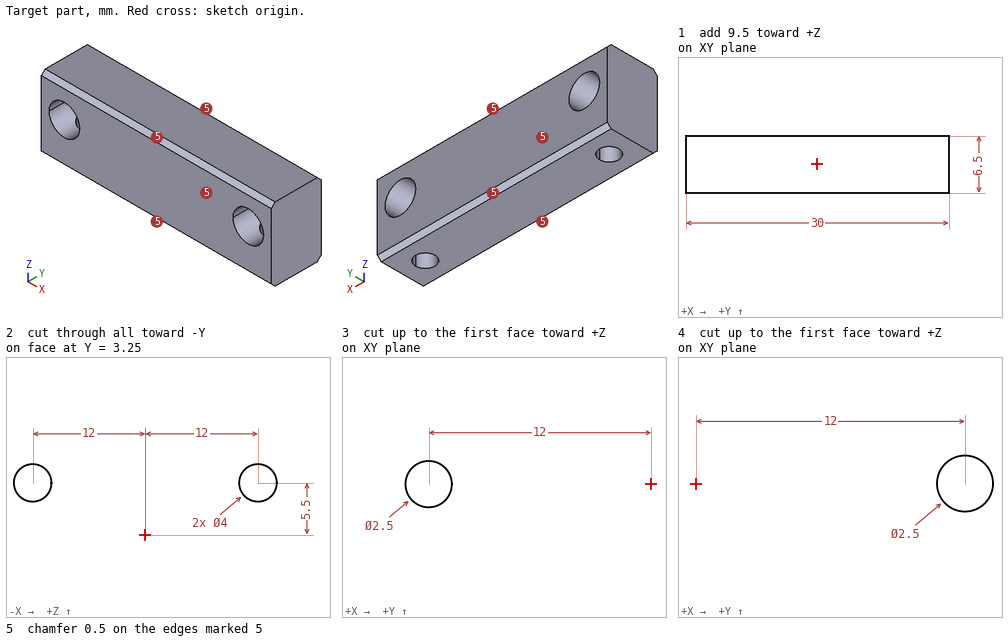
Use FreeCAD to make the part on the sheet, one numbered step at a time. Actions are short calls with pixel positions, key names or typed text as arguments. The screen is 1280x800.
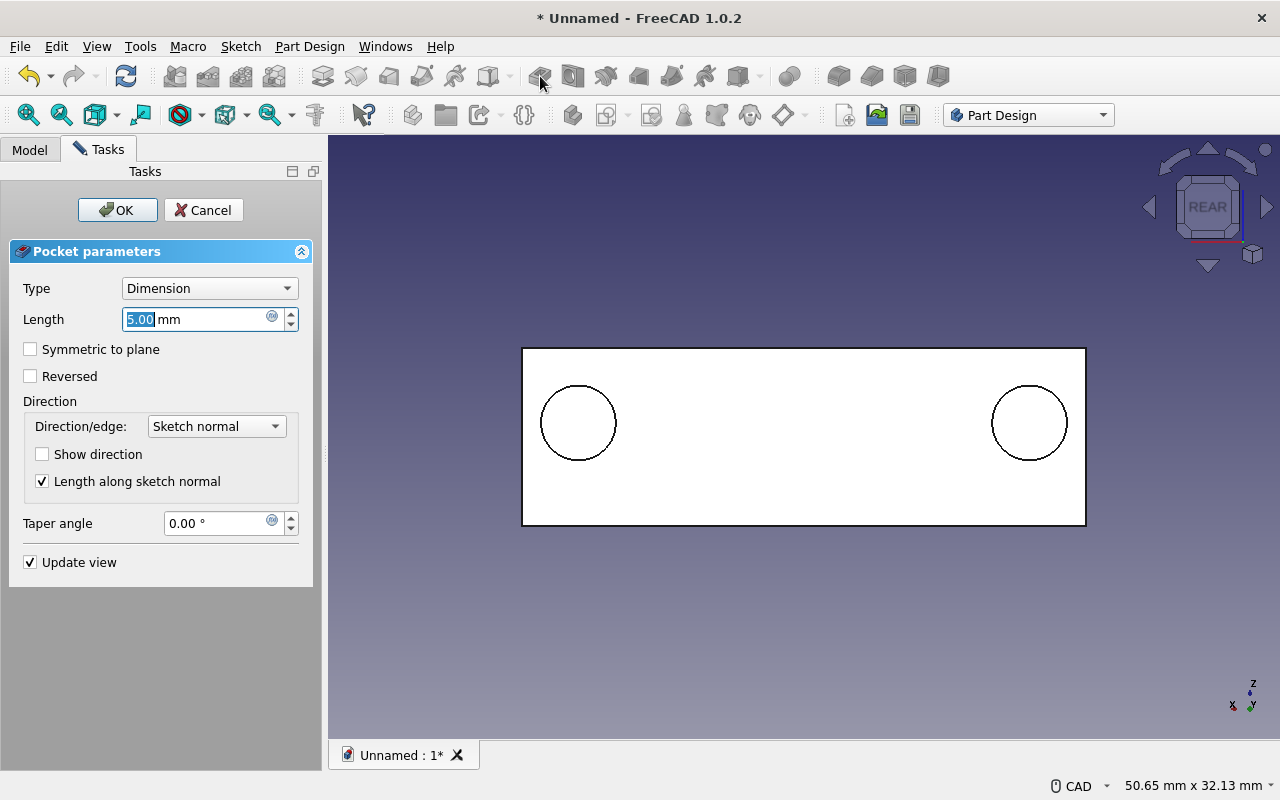
click(210, 288)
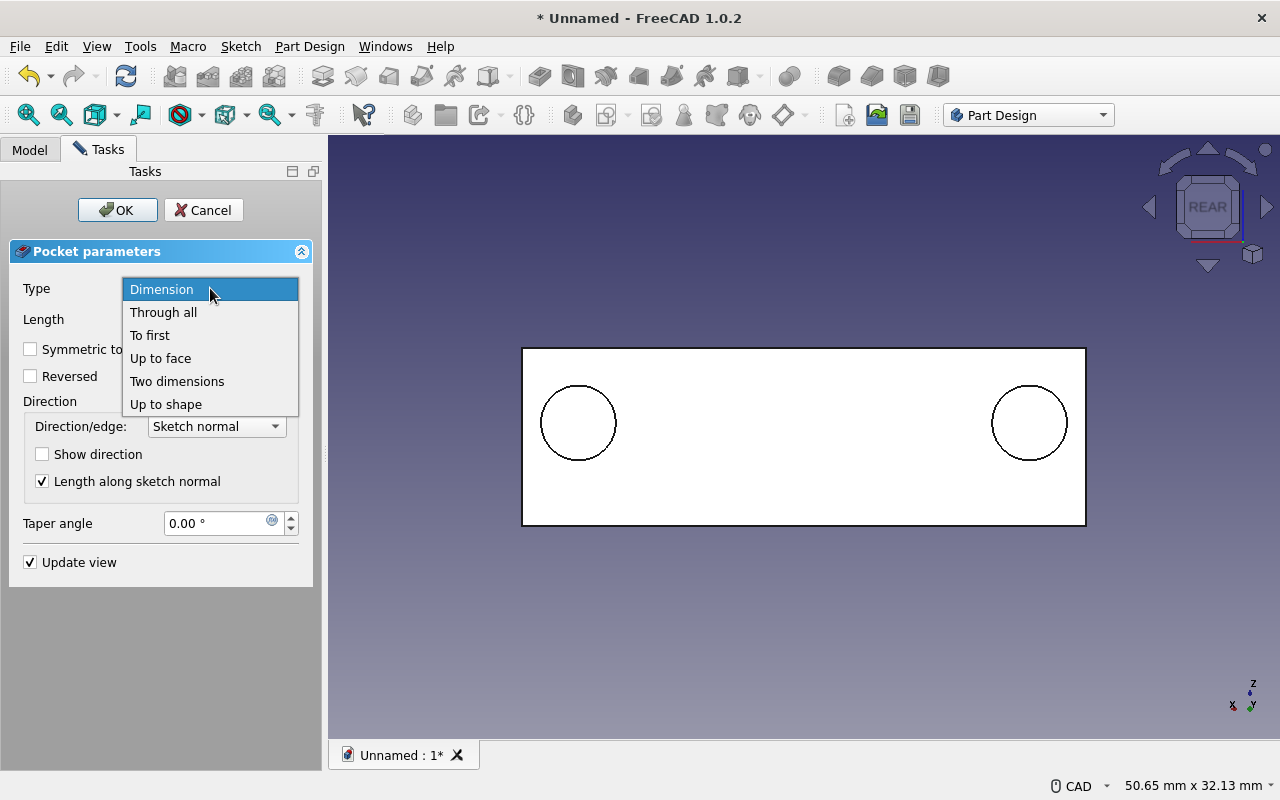
click(208, 312)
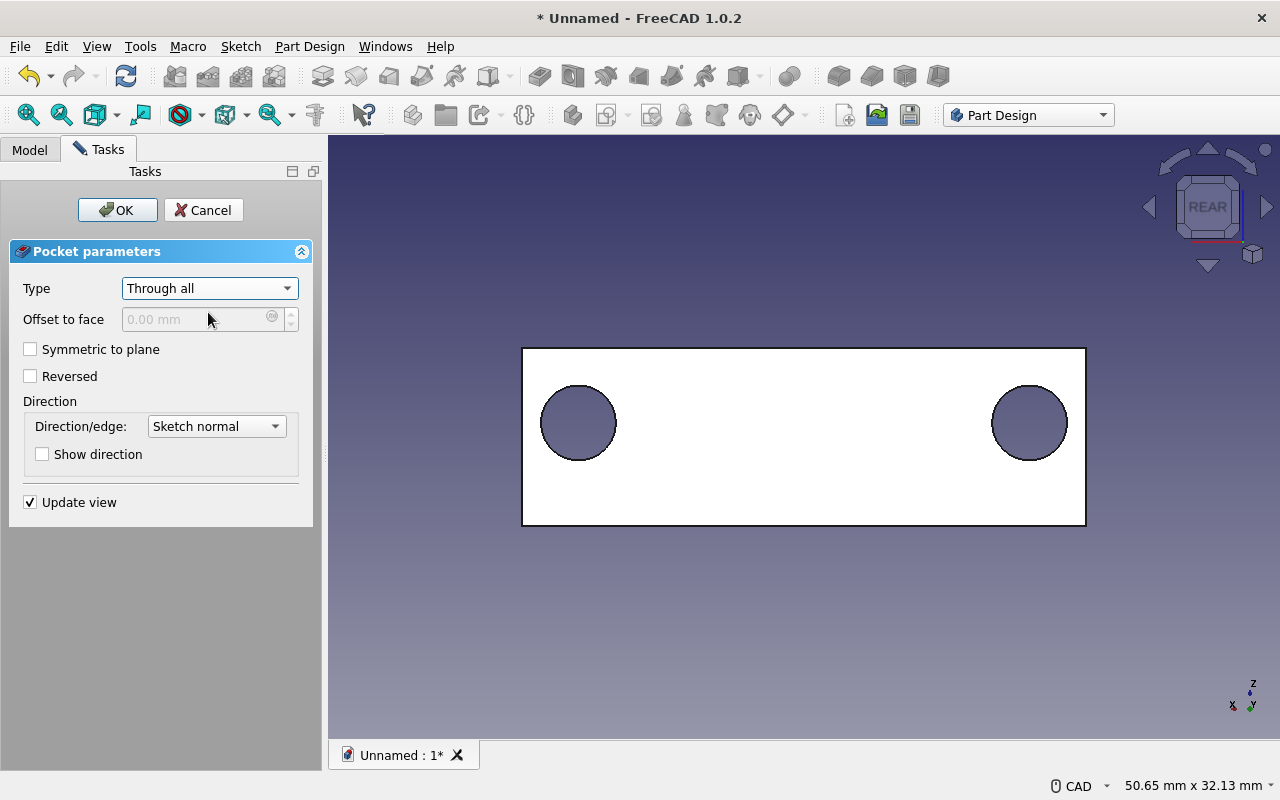
click(118, 210)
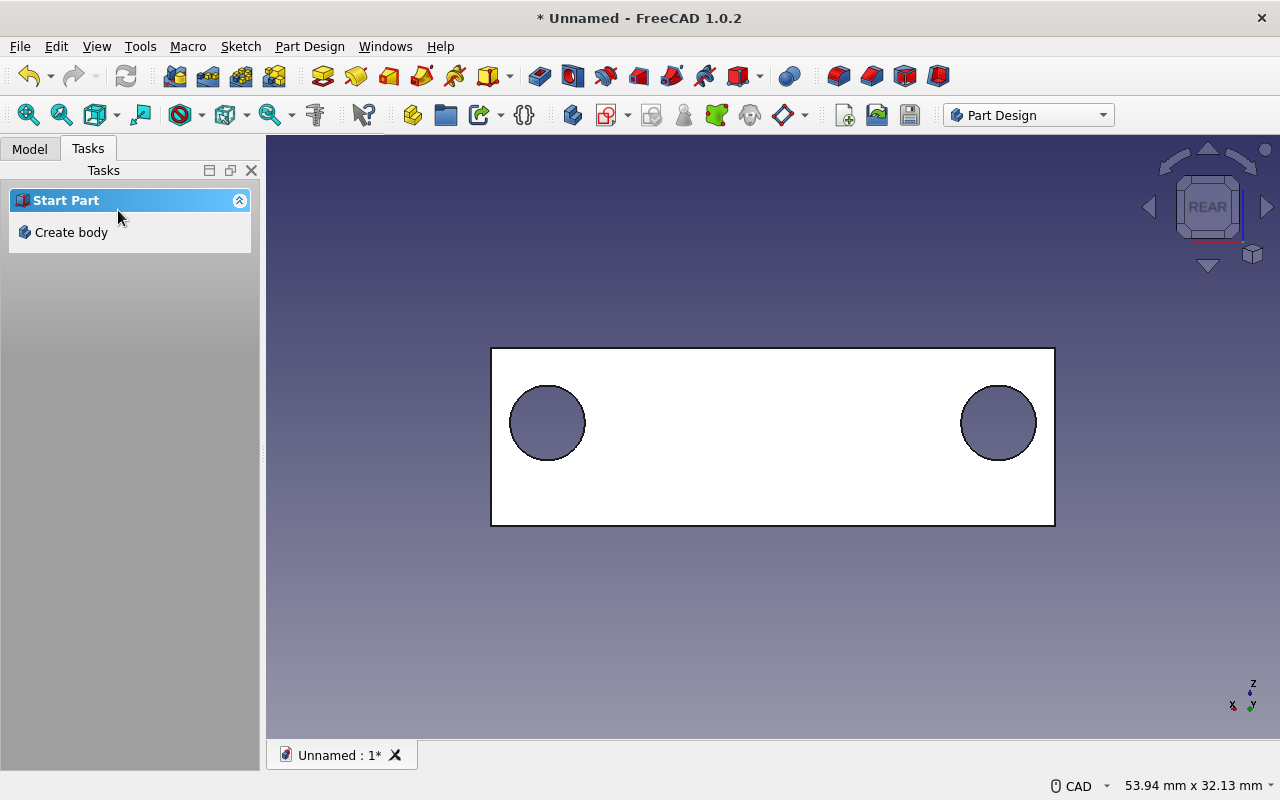
click(606, 116)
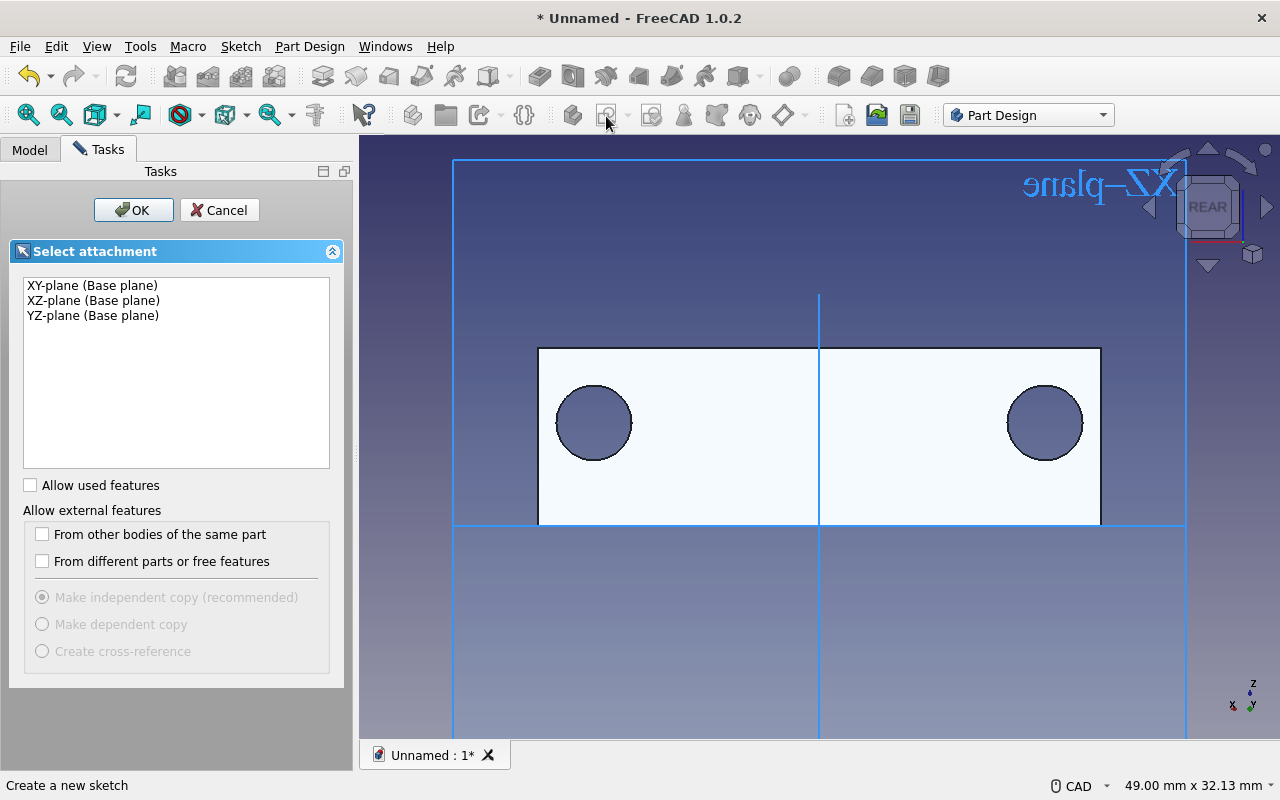
click(84, 286)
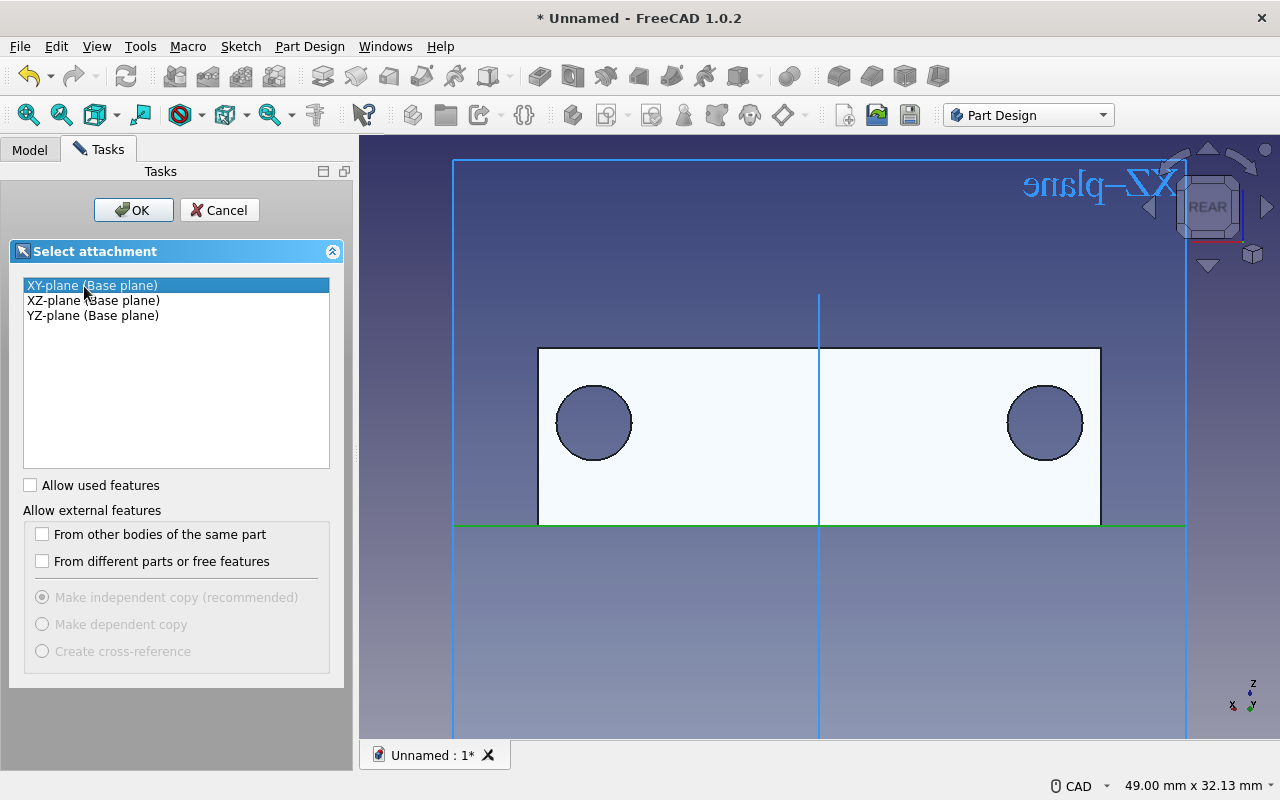
click(134, 210)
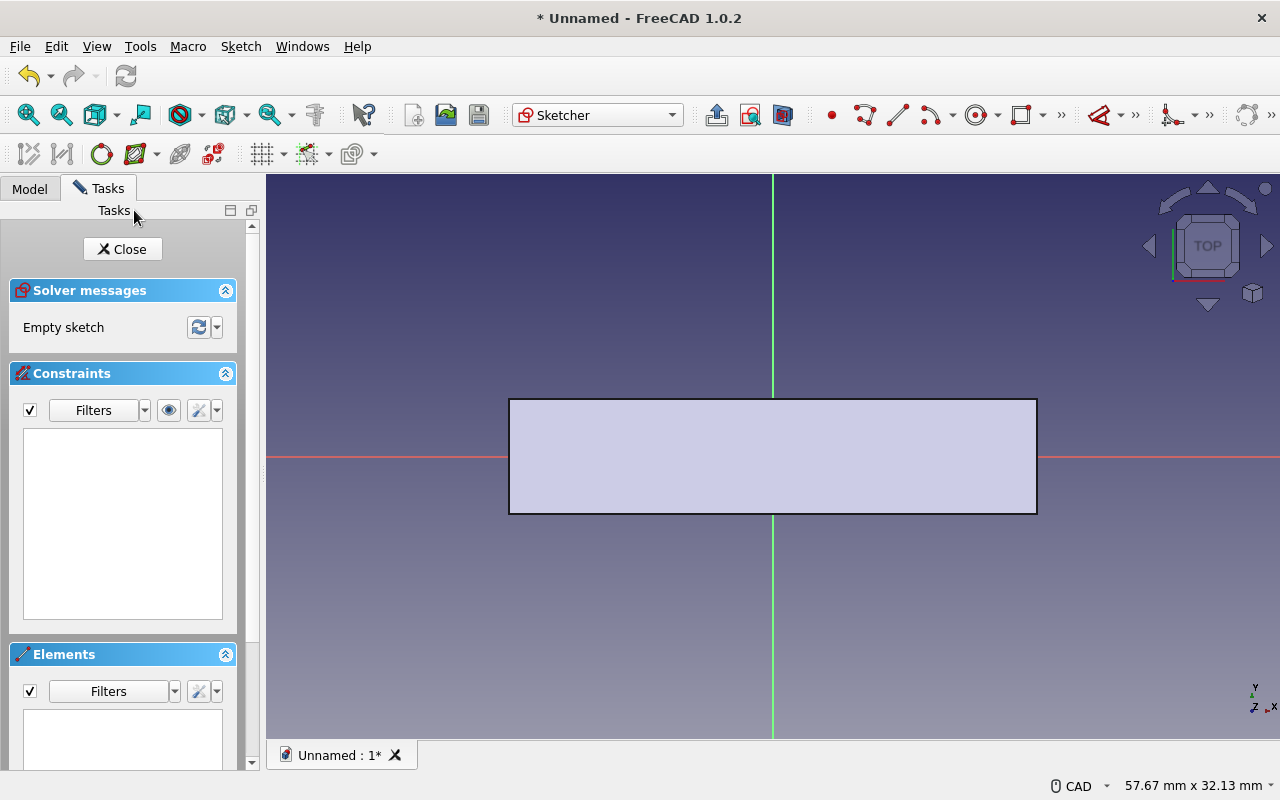
key(q)
key(s)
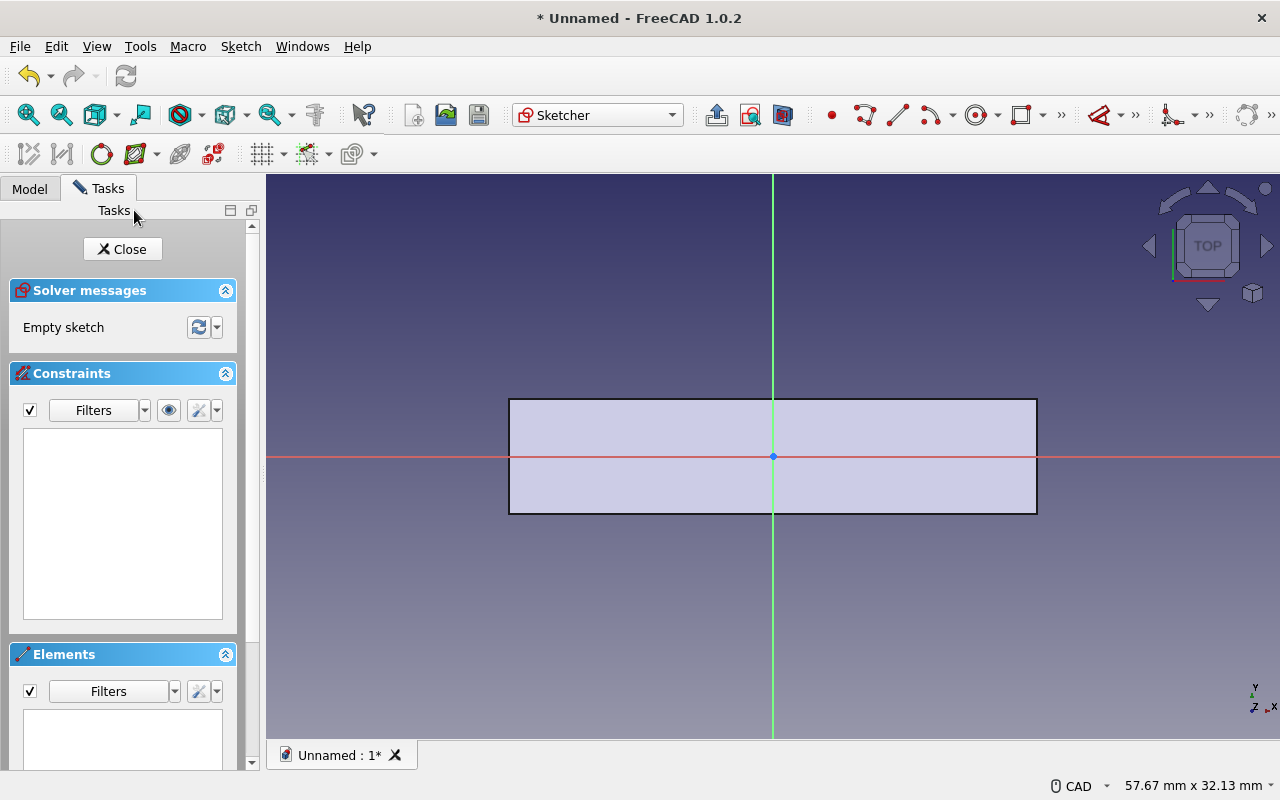
scroll(544, 456, up, 11)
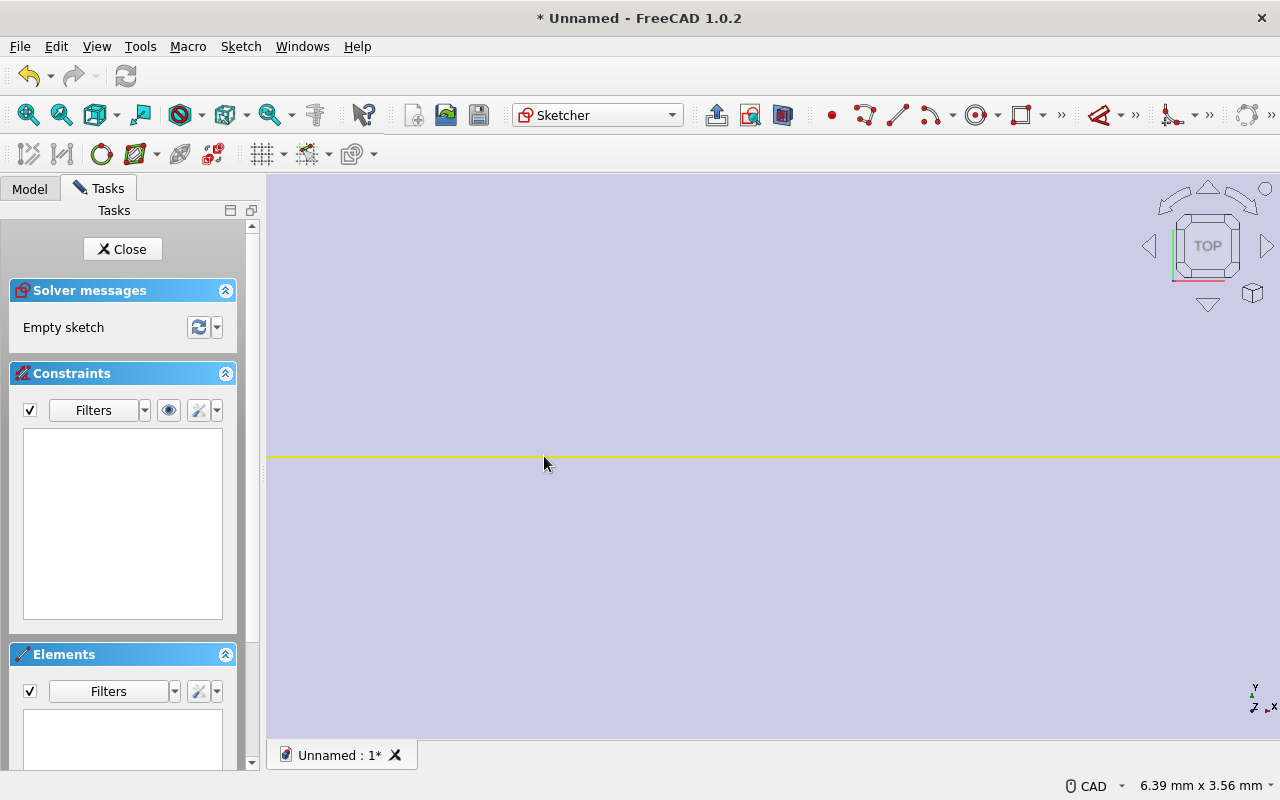
click(976, 116)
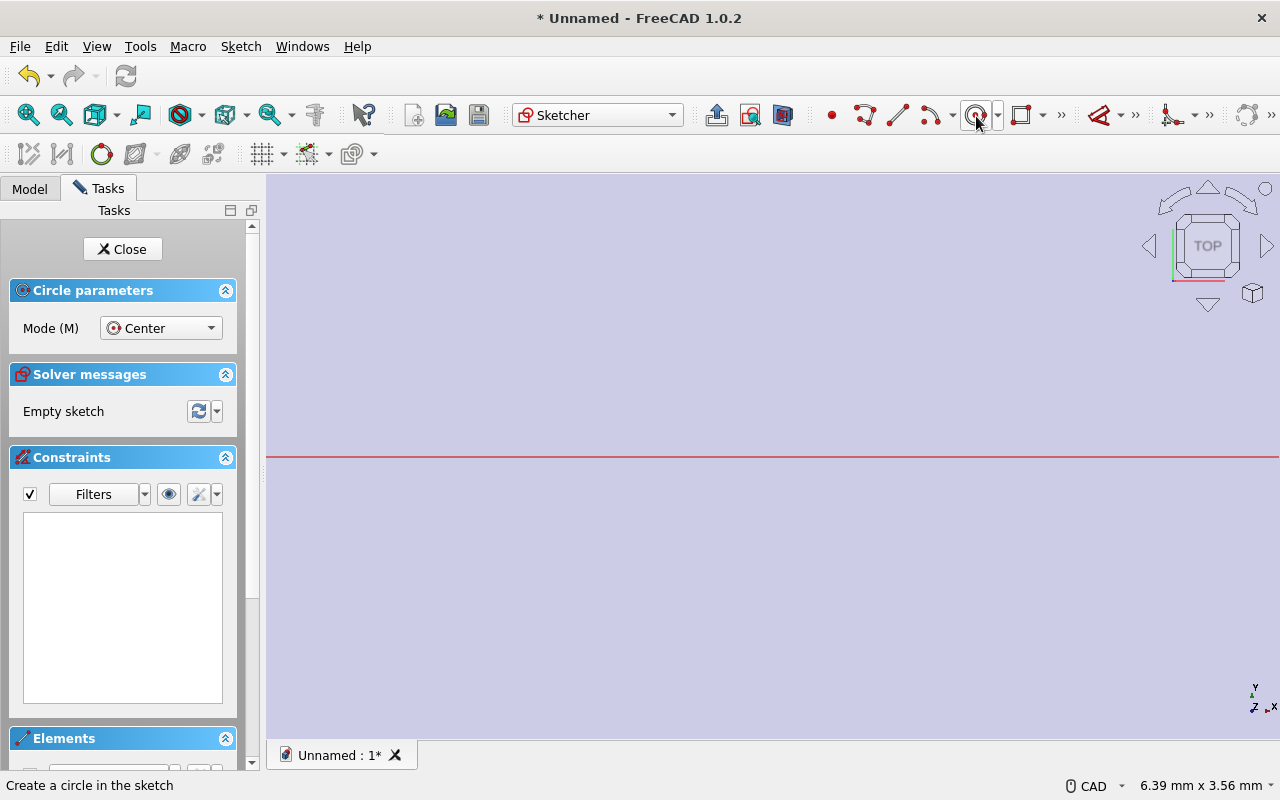
click(704, 456)
click(845, 316)
key(Escape)